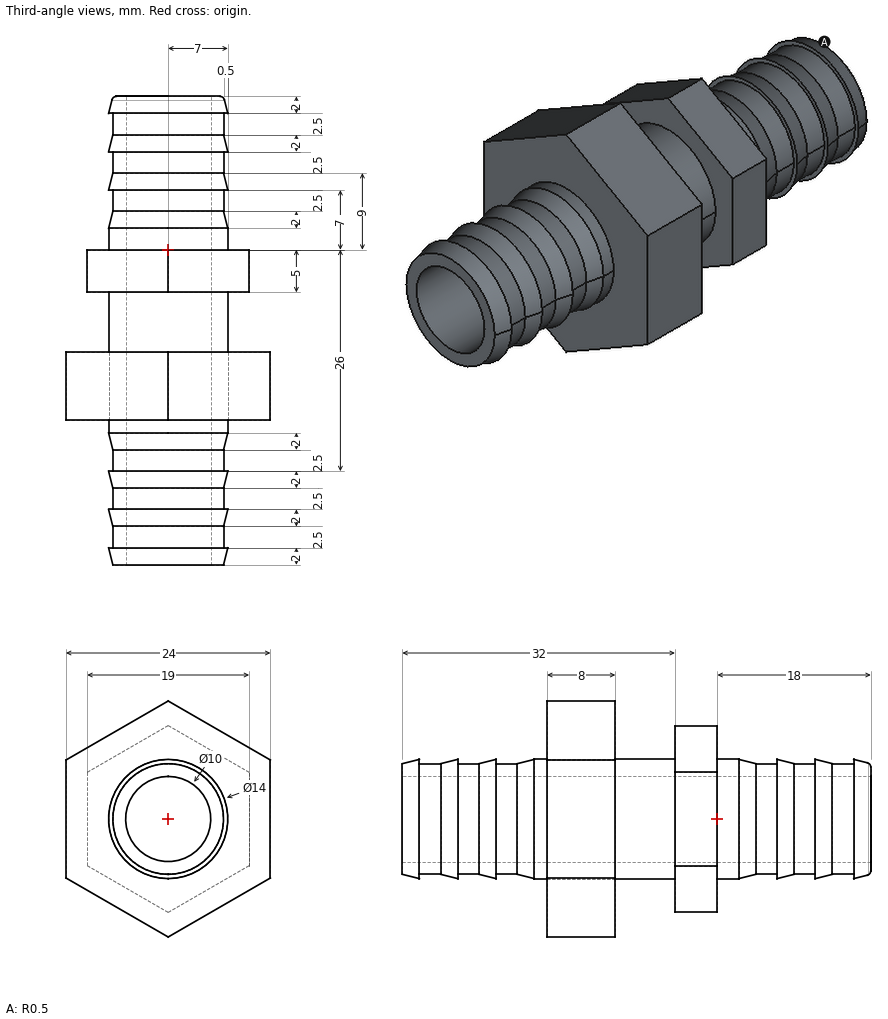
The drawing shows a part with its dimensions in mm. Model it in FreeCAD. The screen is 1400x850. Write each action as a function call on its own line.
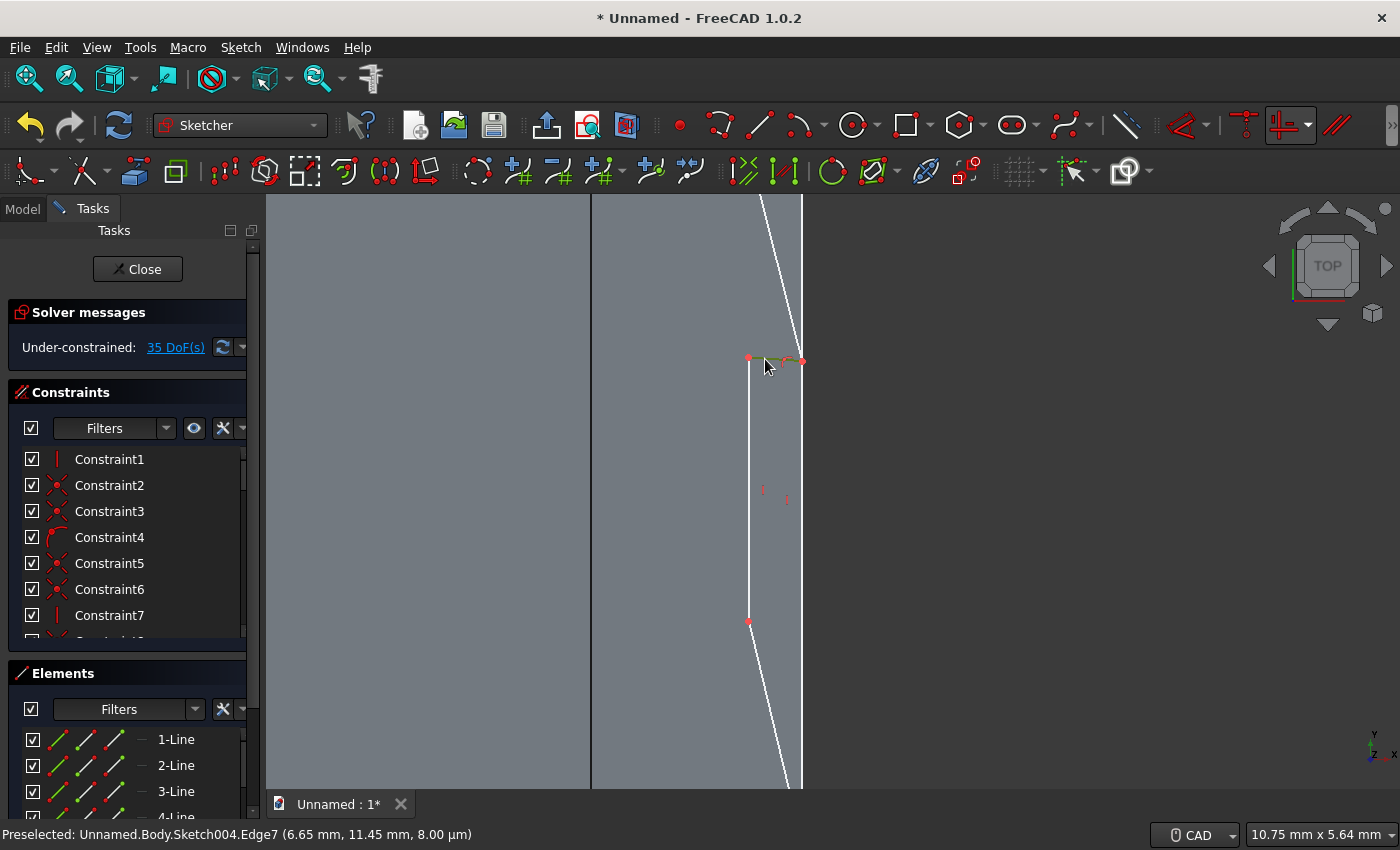
click(1310, 126)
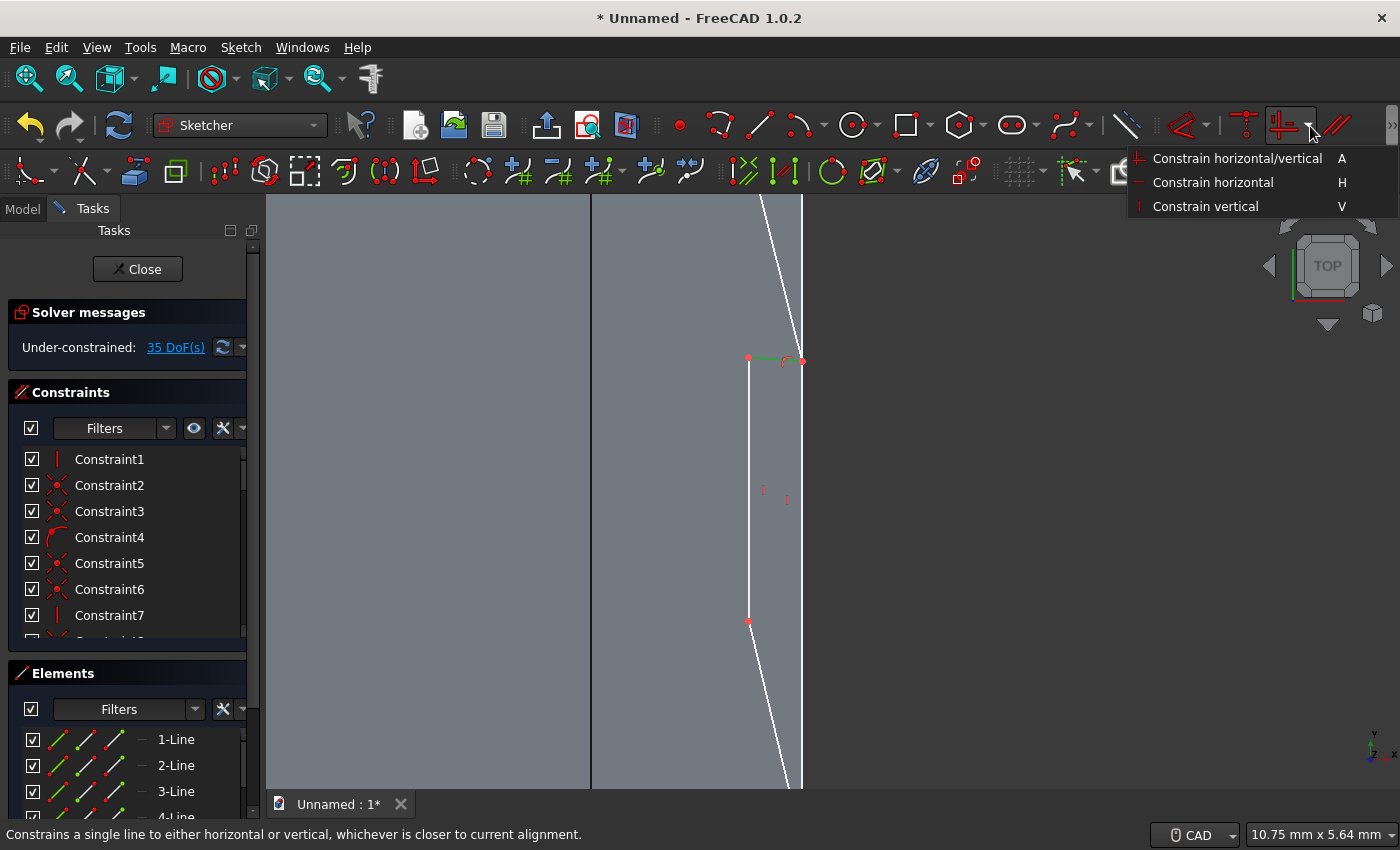
click(1263, 182)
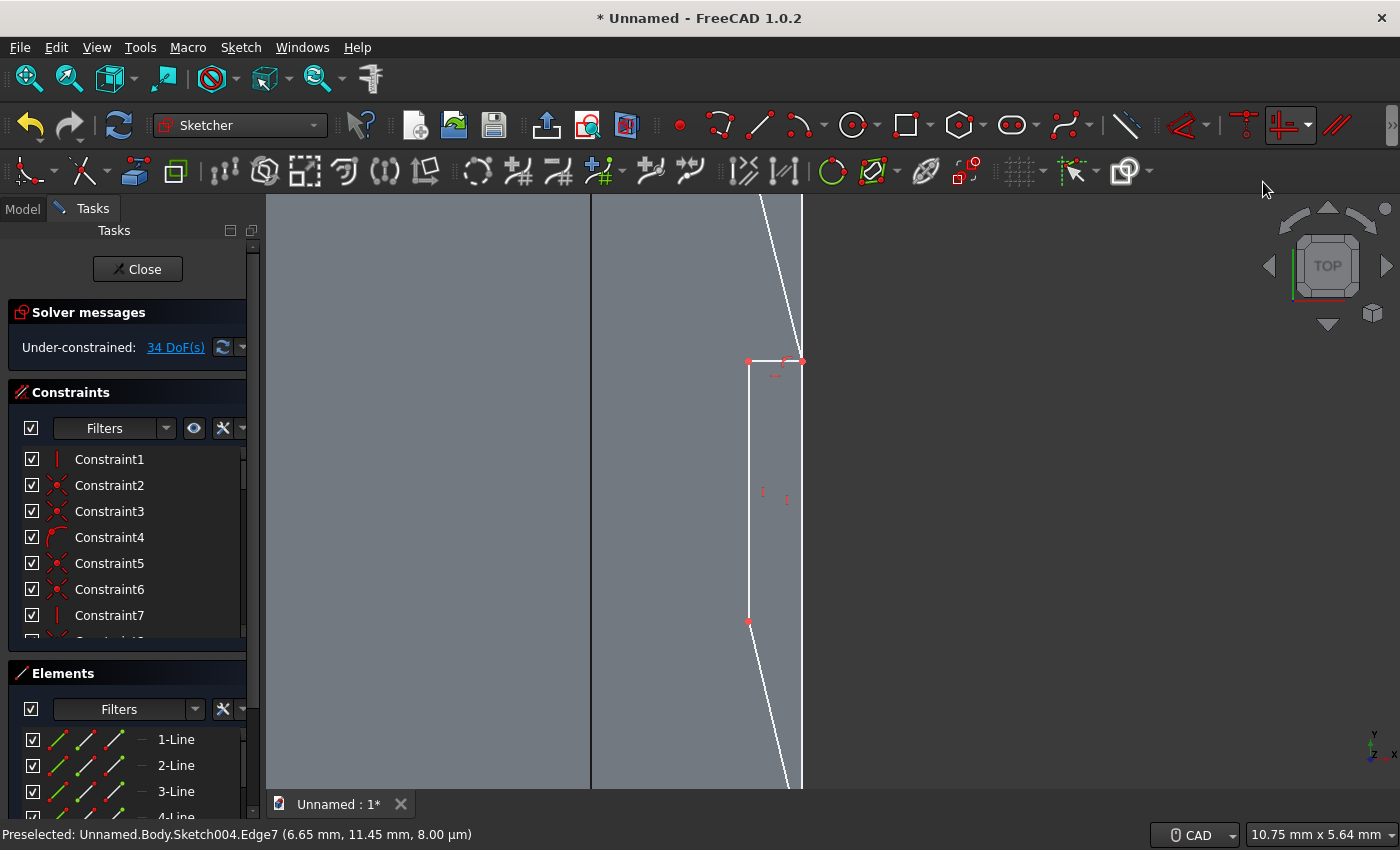
scroll(786, 357, down, 14)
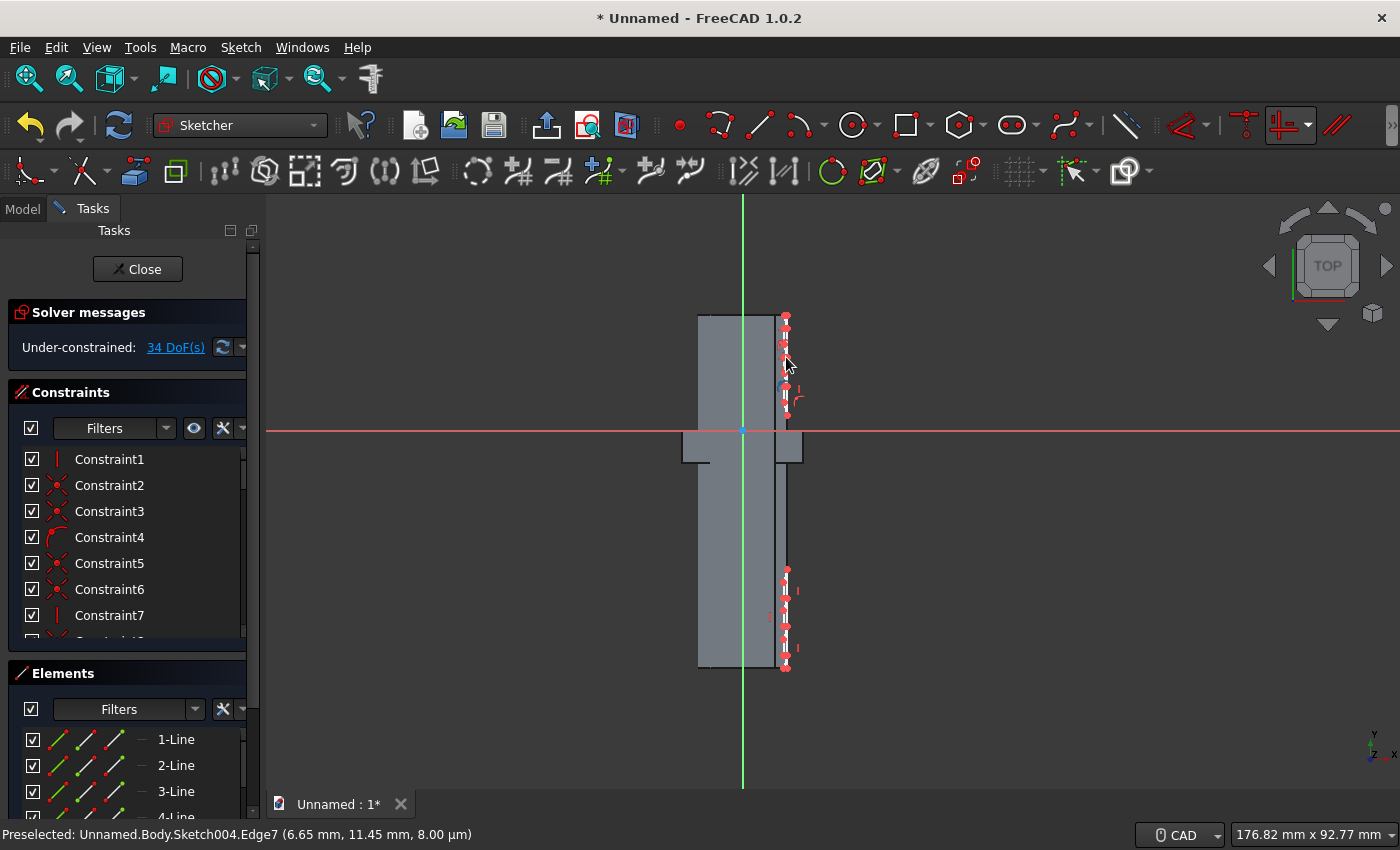
scroll(786, 387, up, 14)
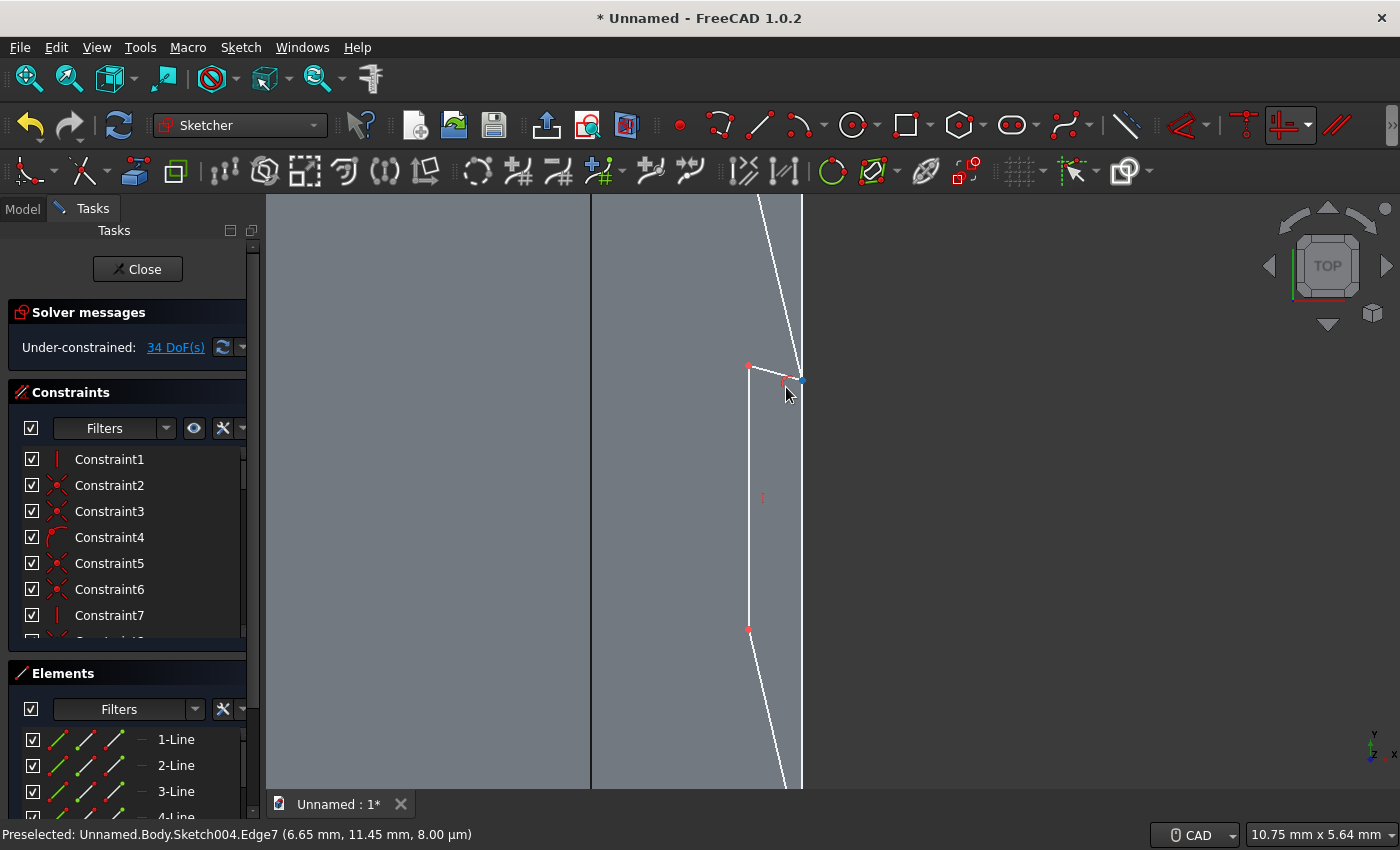
click(765, 370)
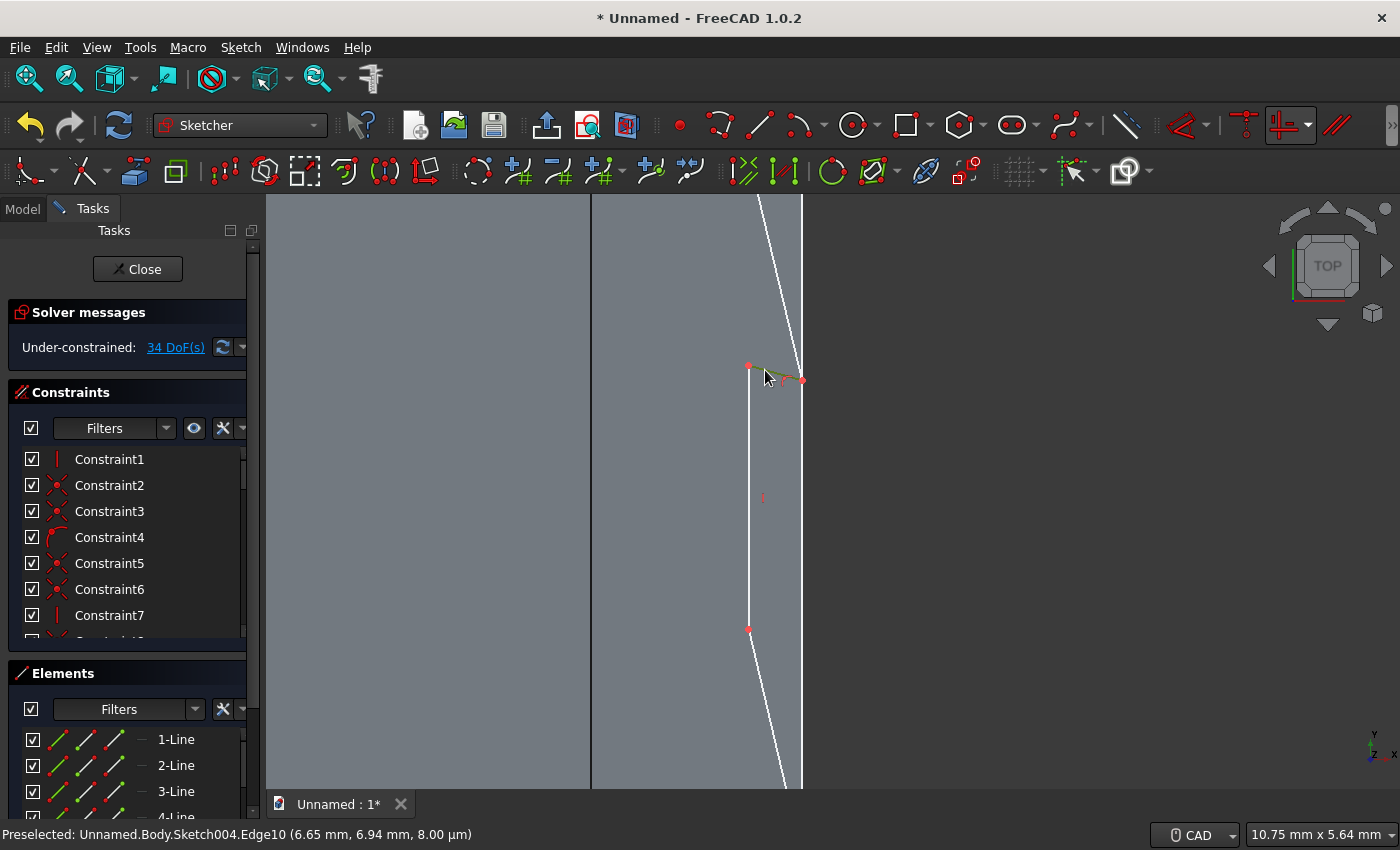
click(1310, 126)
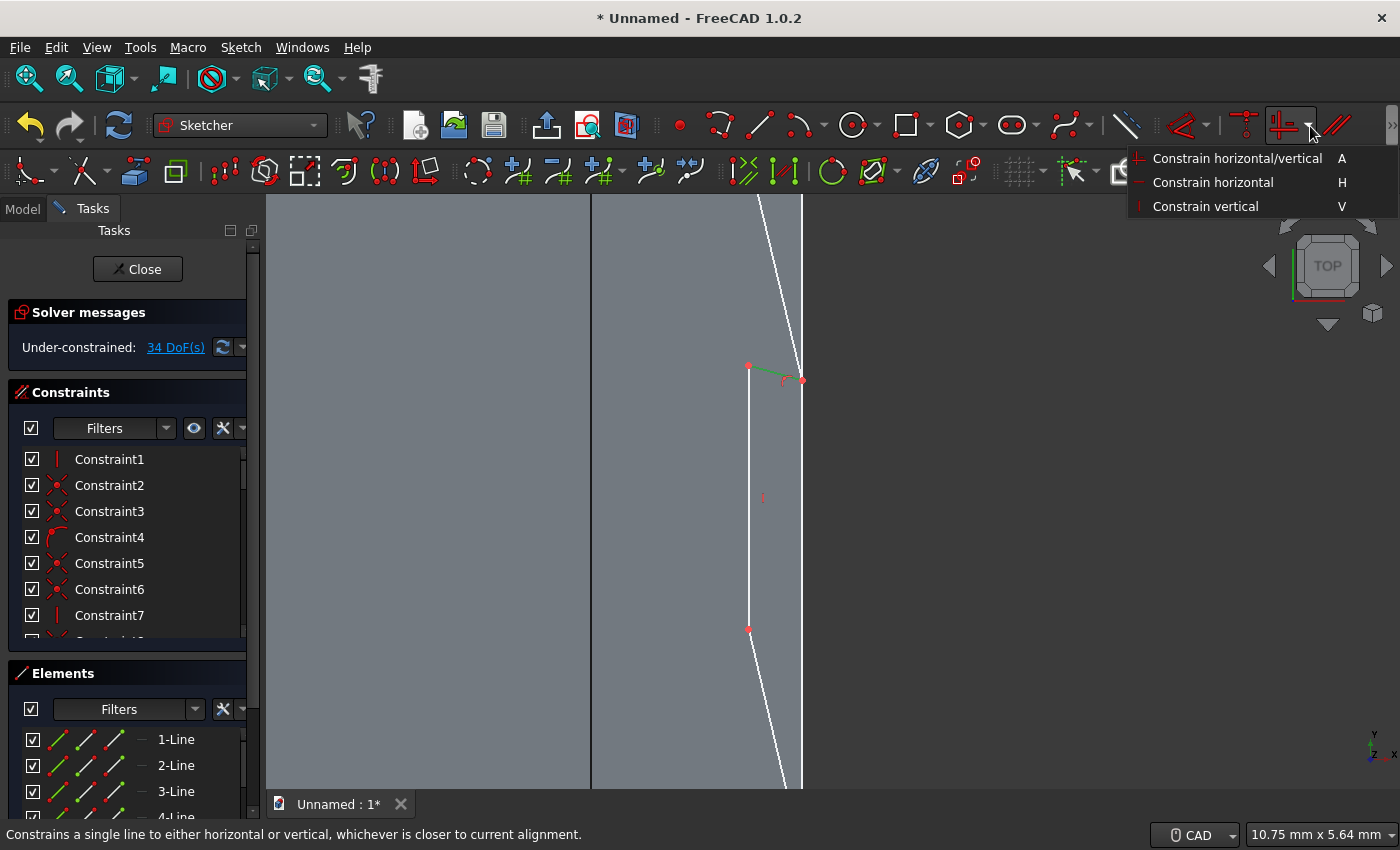
click(1263, 182)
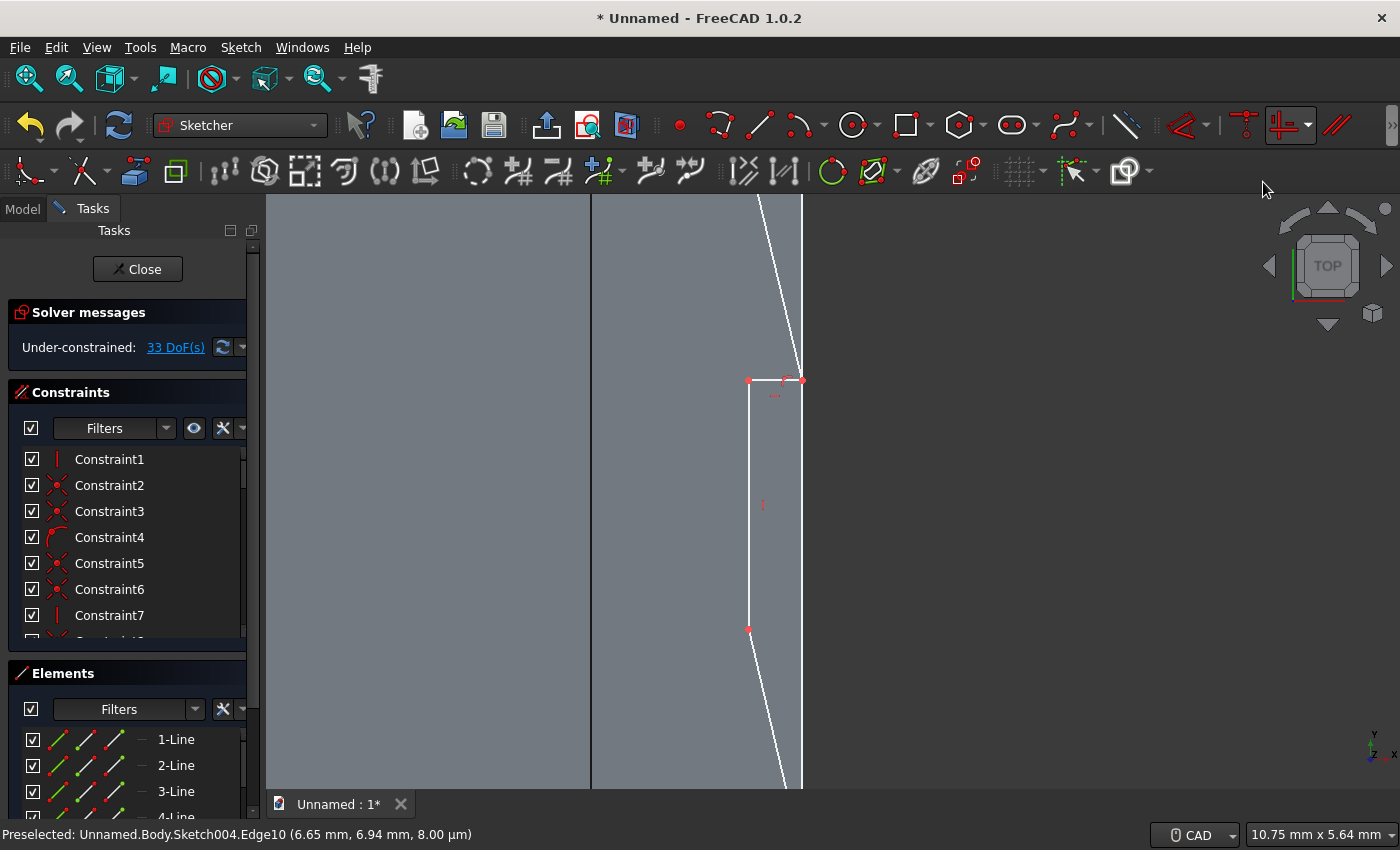
scroll(786, 387, down, 14)